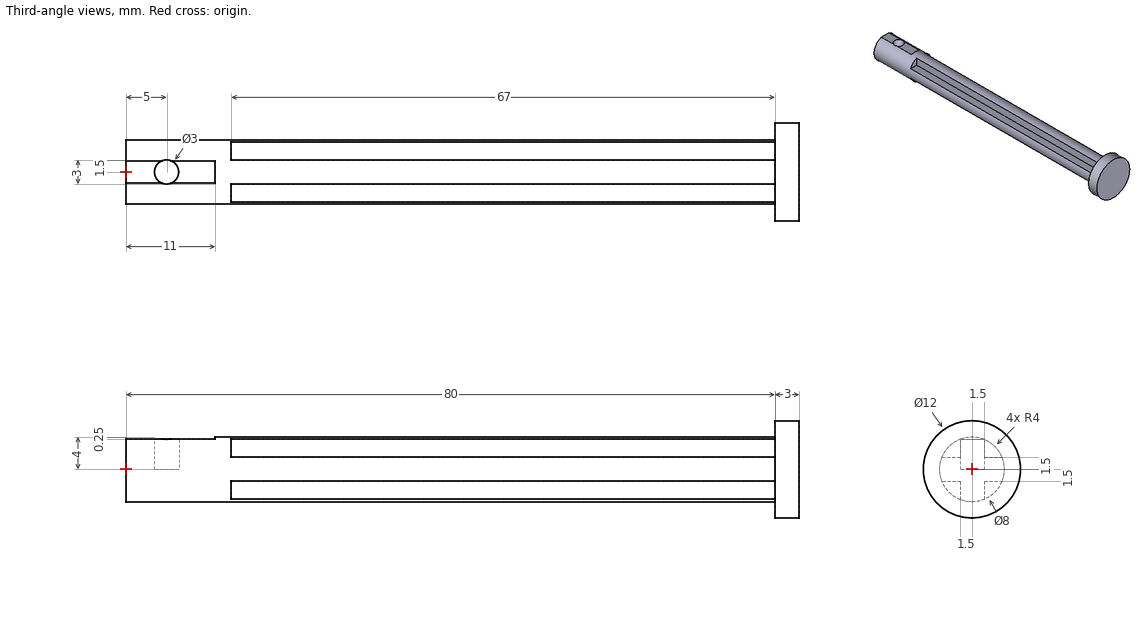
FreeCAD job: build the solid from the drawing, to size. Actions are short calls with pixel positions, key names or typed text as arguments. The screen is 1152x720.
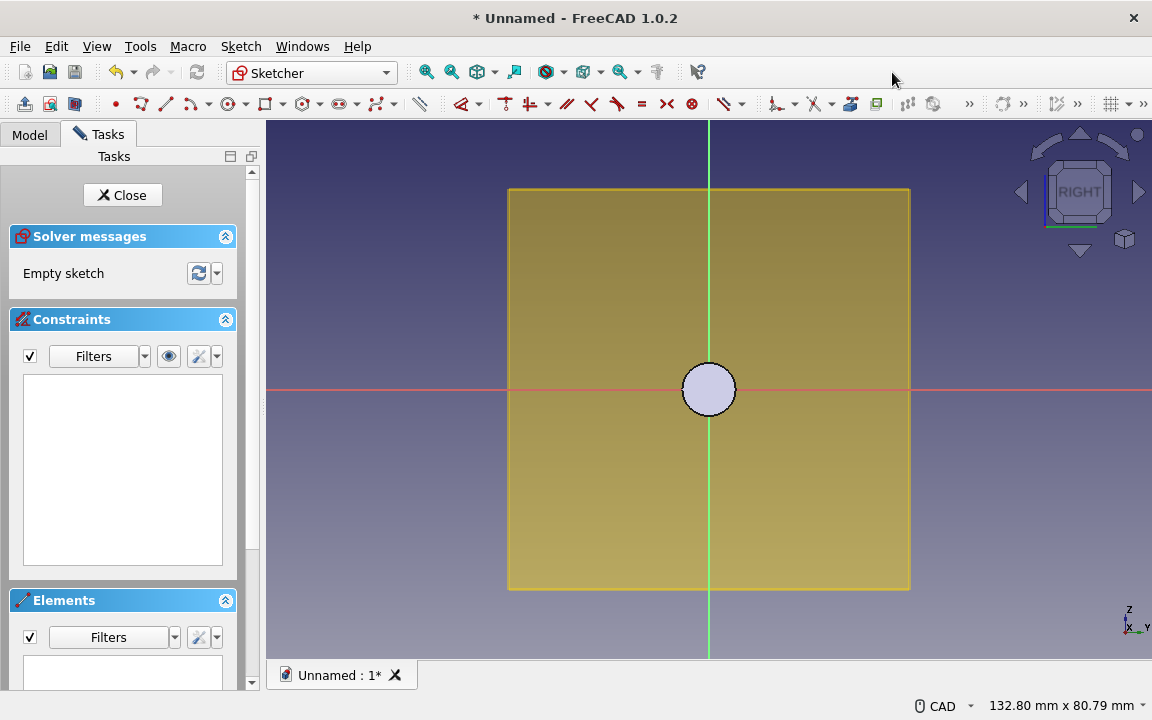
key(q)
key(s)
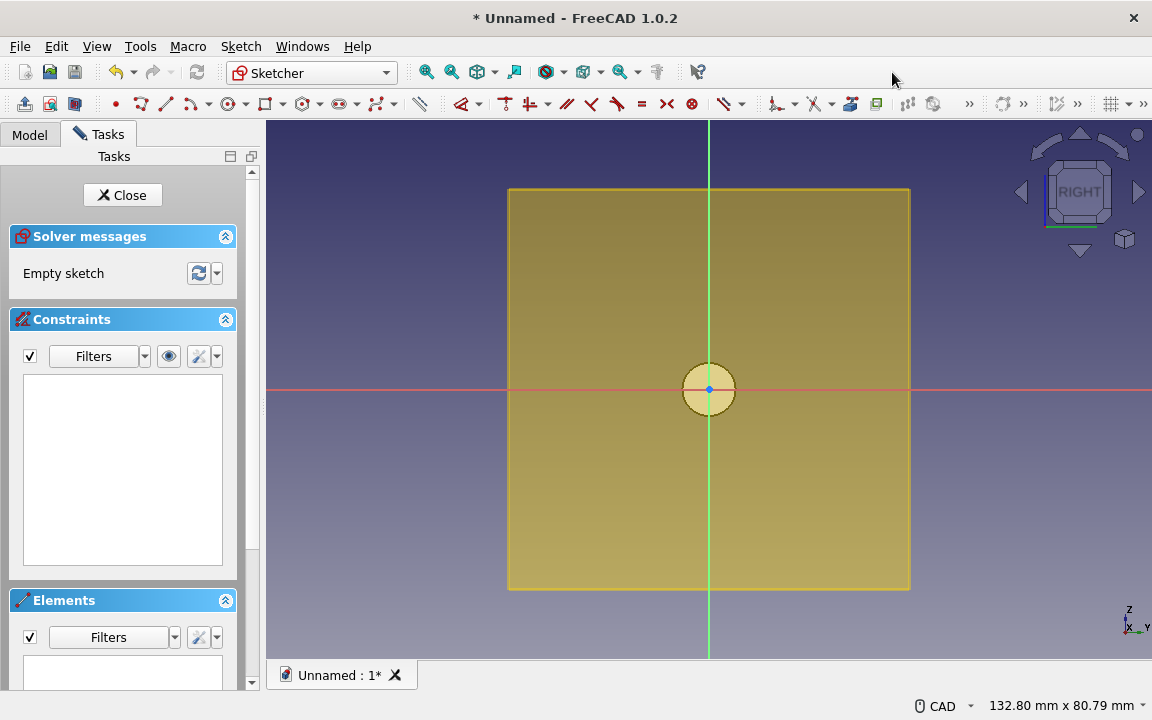
scroll(720, 390, up, 10)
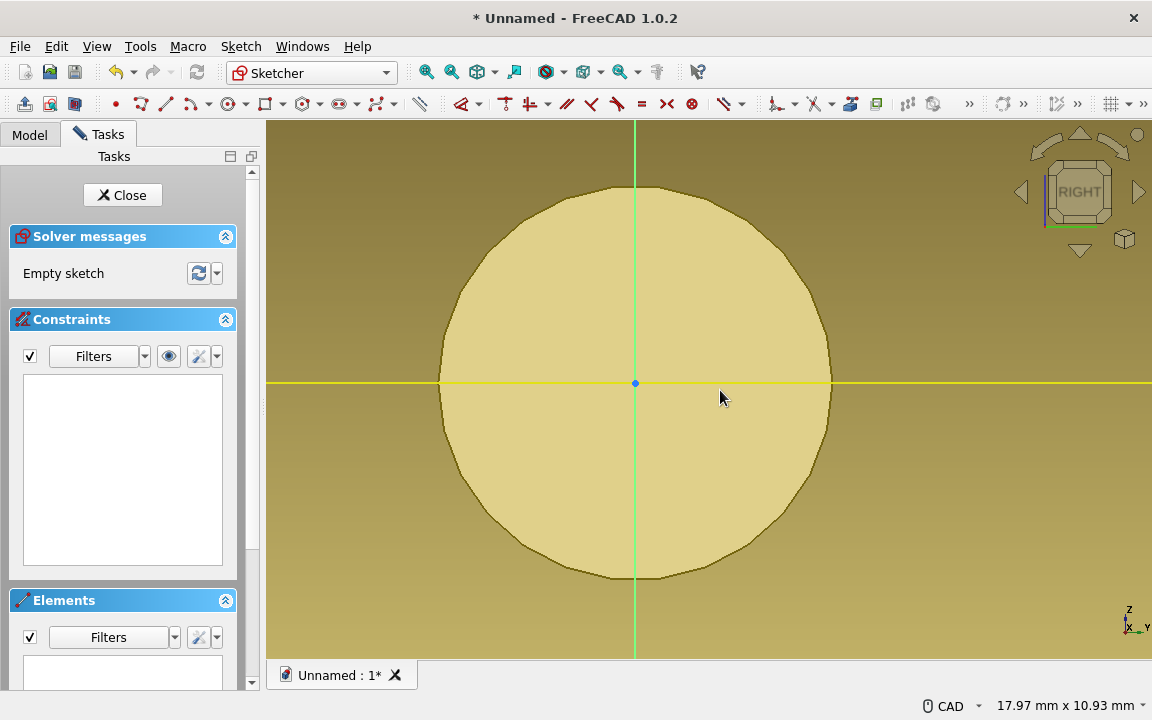
key(g)
key(m)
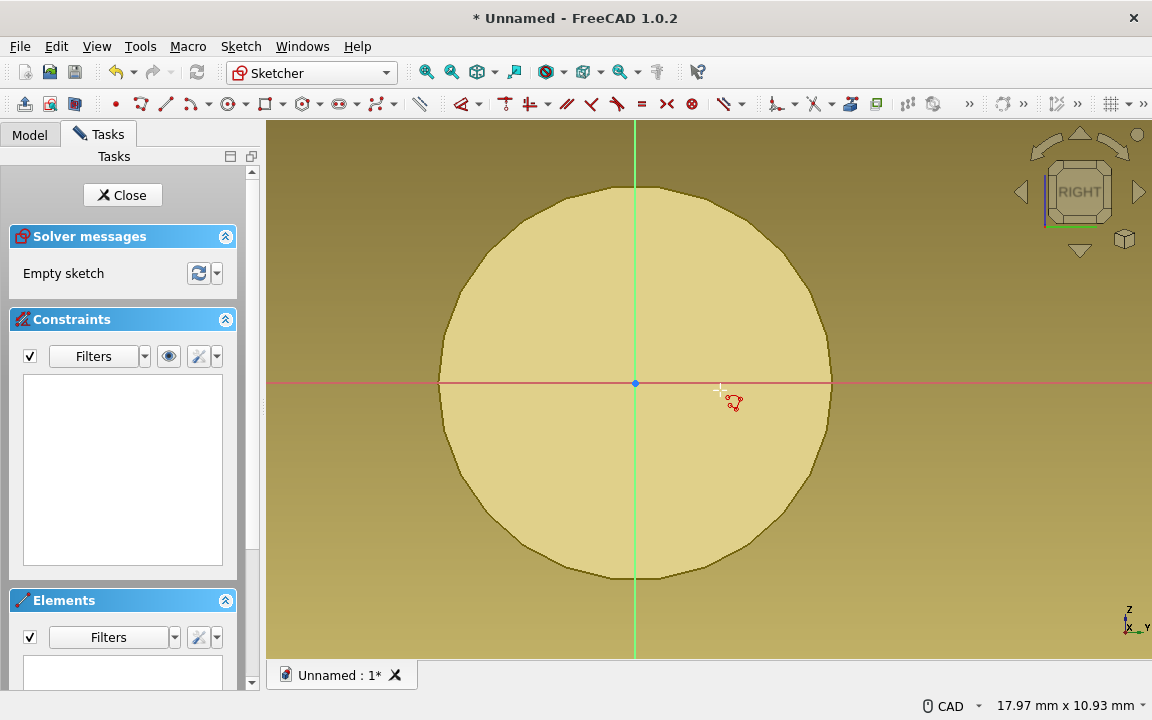
click(709, 200)
click(709, 309)
click(818, 309)
right_click(818, 309)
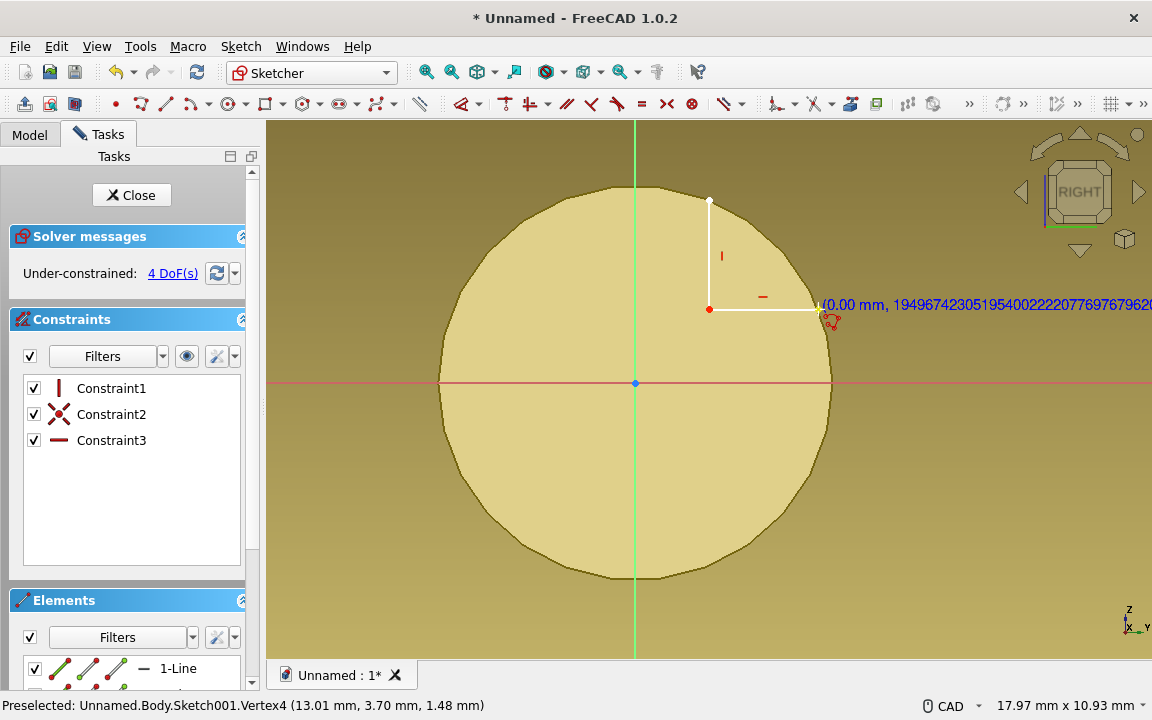
key(g)
key(3)
key(a)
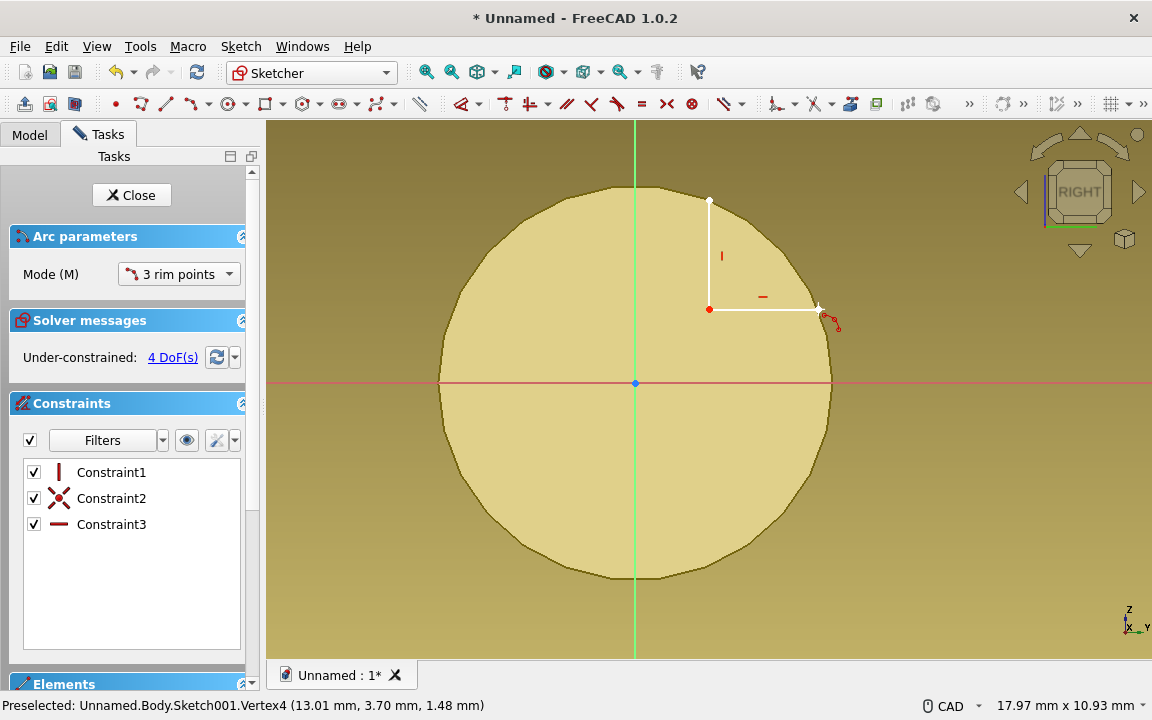
click(818, 310)
click(709, 201)
click(775, 244)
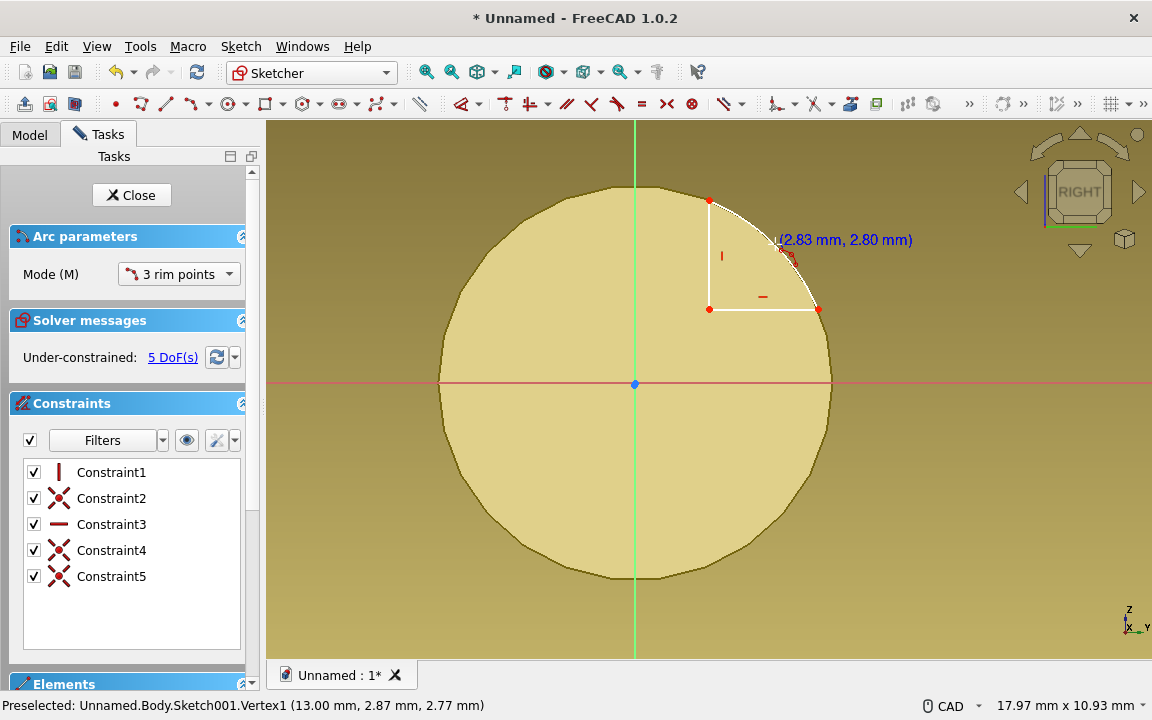
key(g)
key(m)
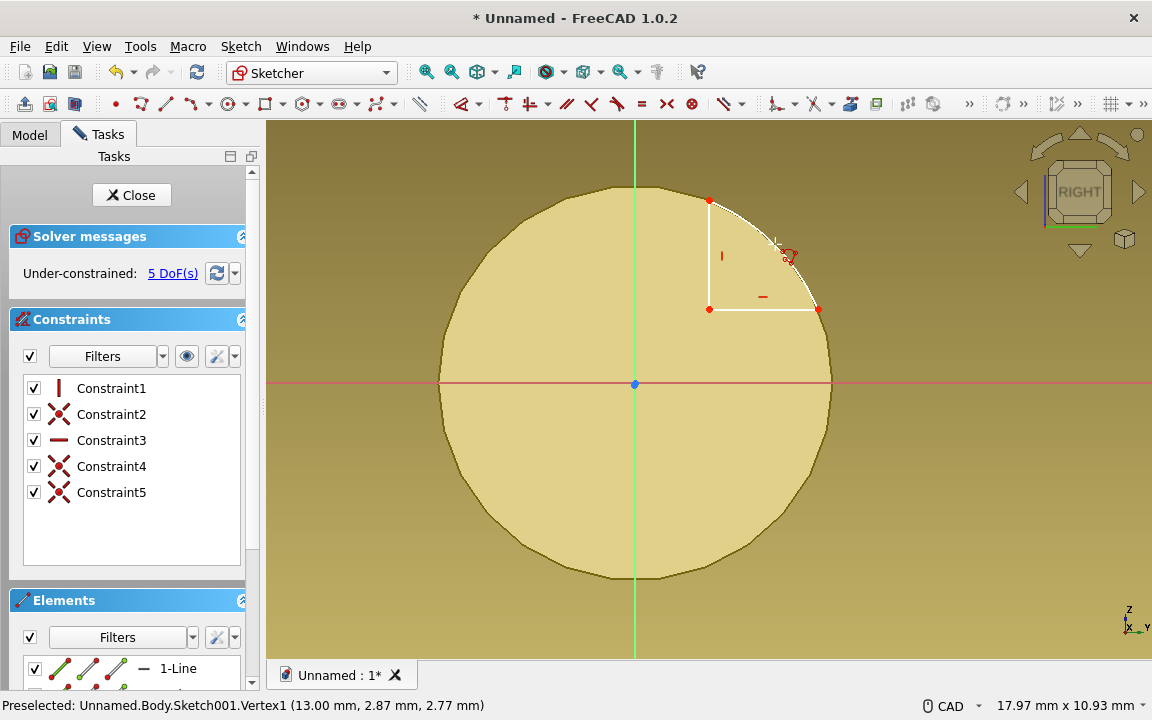
click(818, 457)
click(709, 457)
click(709, 566)
right_click(709, 566)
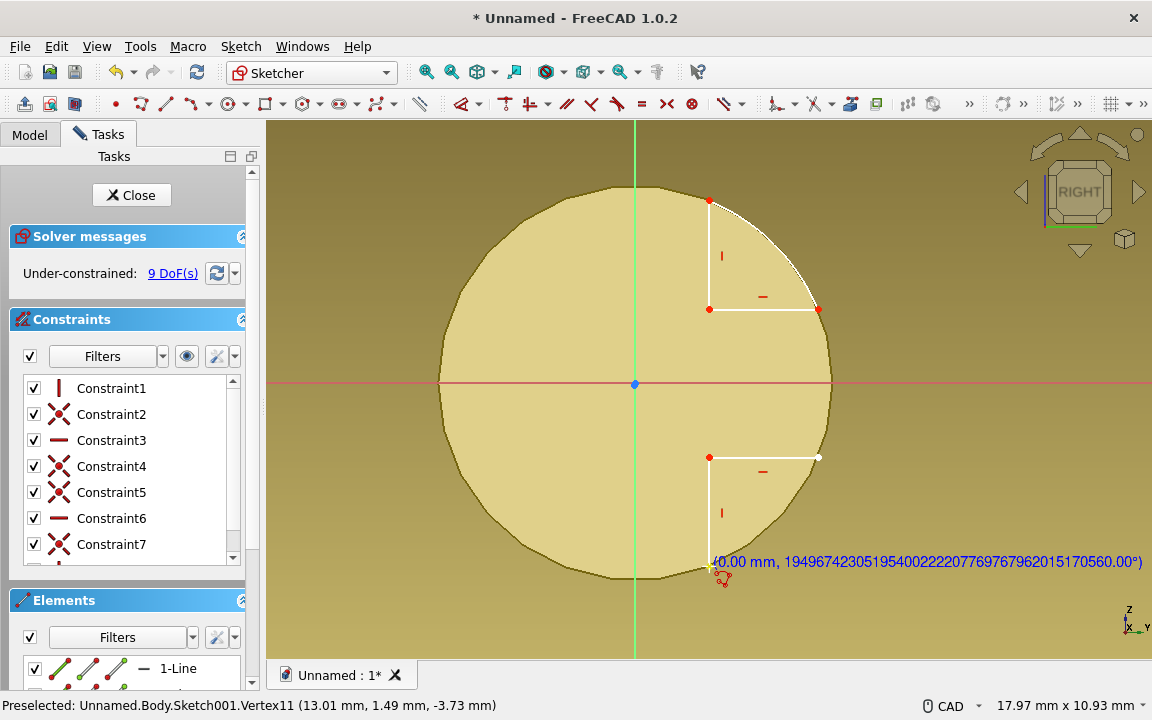
key(g)
key(3)
key(a)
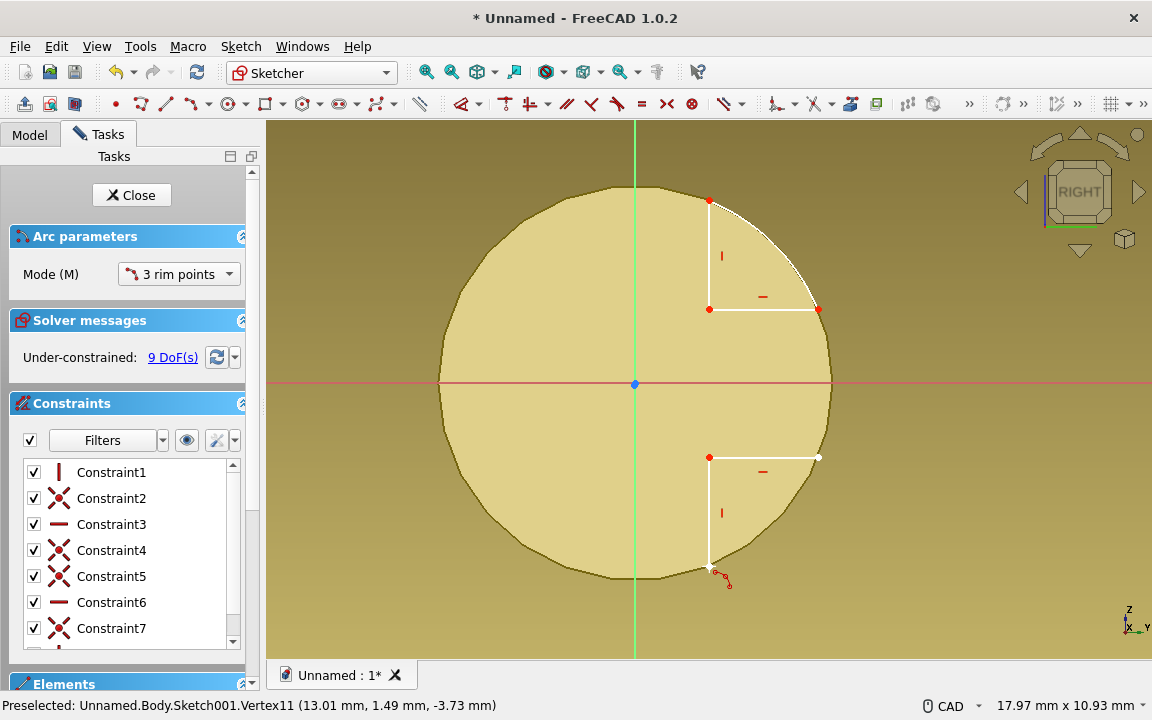
click(709, 567)
click(818, 458)
click(775, 523)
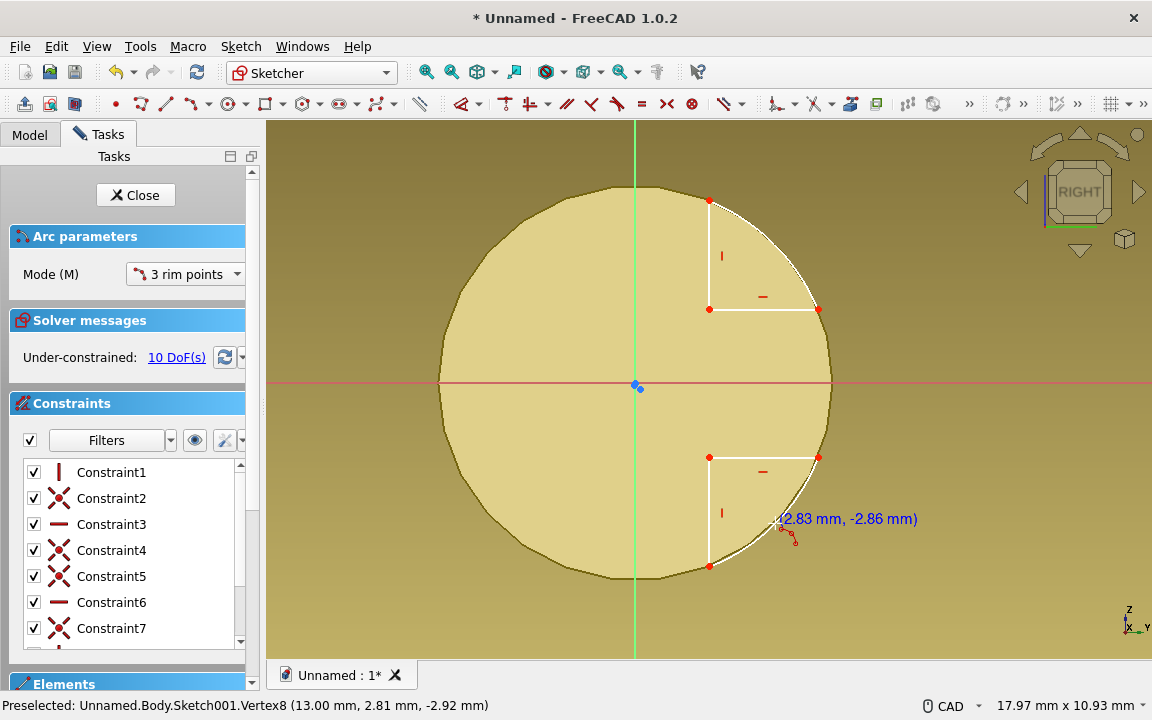
key(g)
key(m)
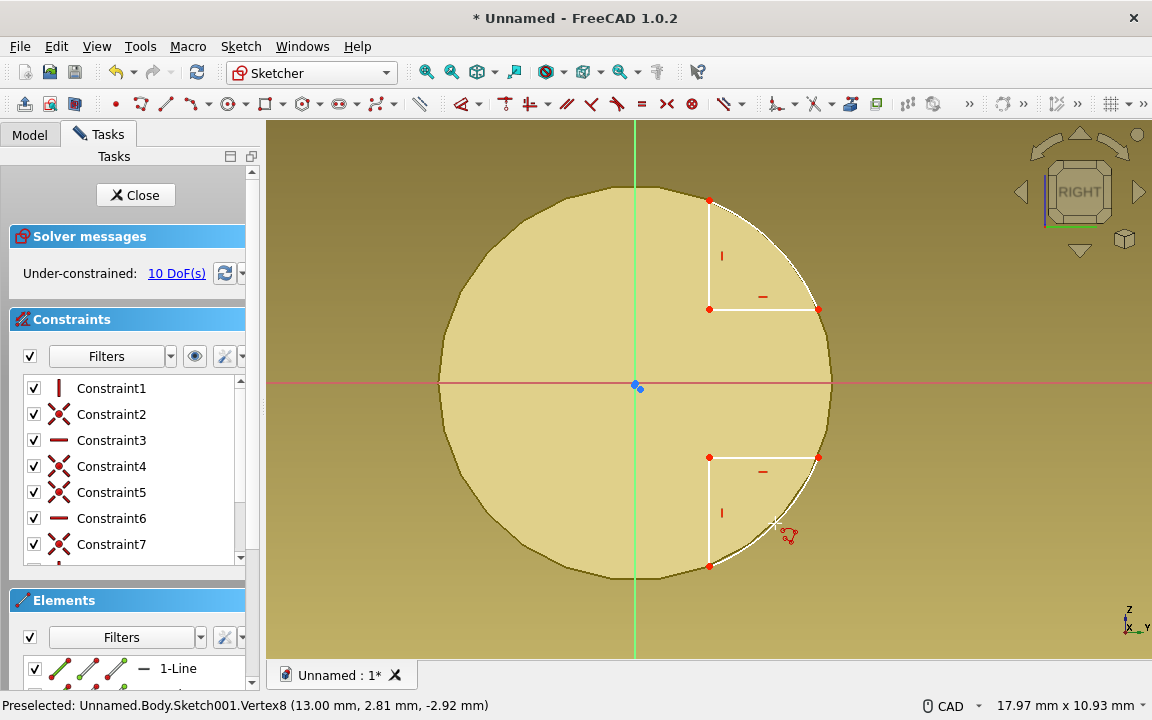
click(561, 566)
click(561, 457)
click(453, 457)
right_click(453, 457)